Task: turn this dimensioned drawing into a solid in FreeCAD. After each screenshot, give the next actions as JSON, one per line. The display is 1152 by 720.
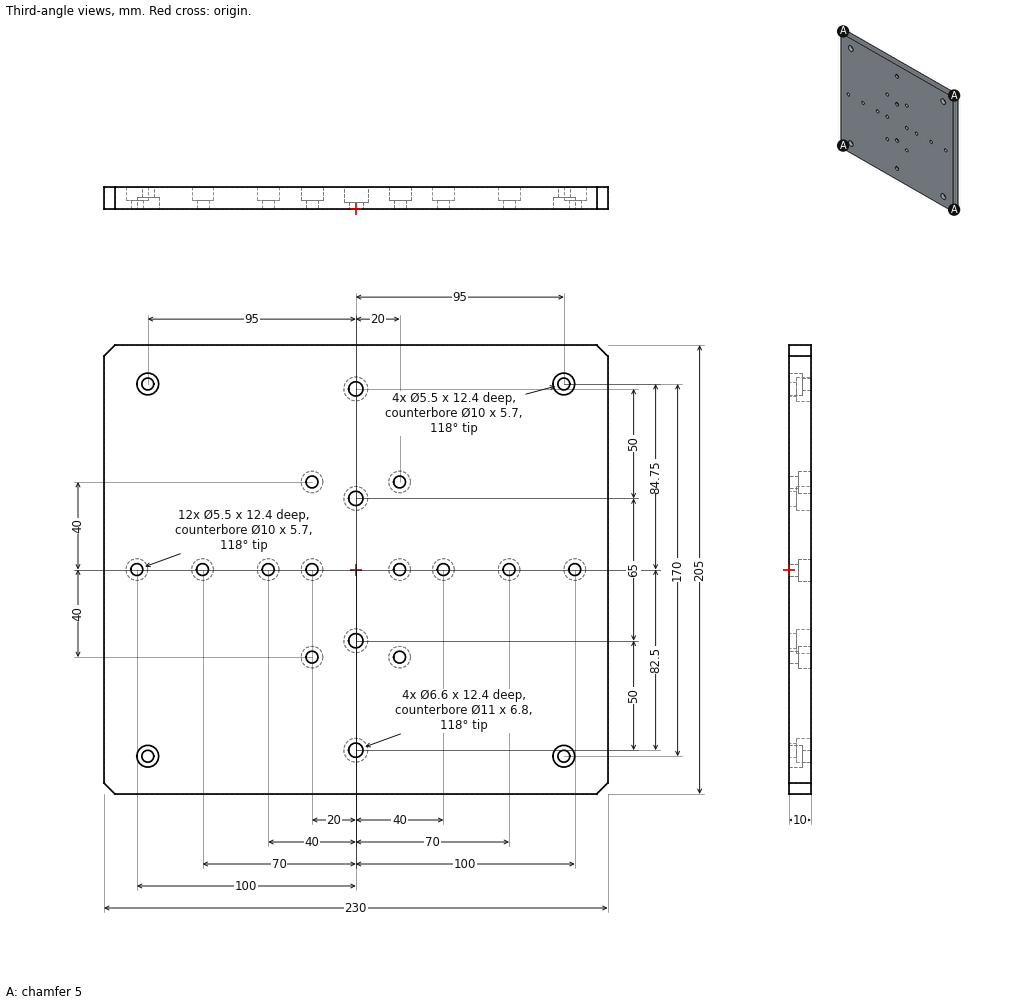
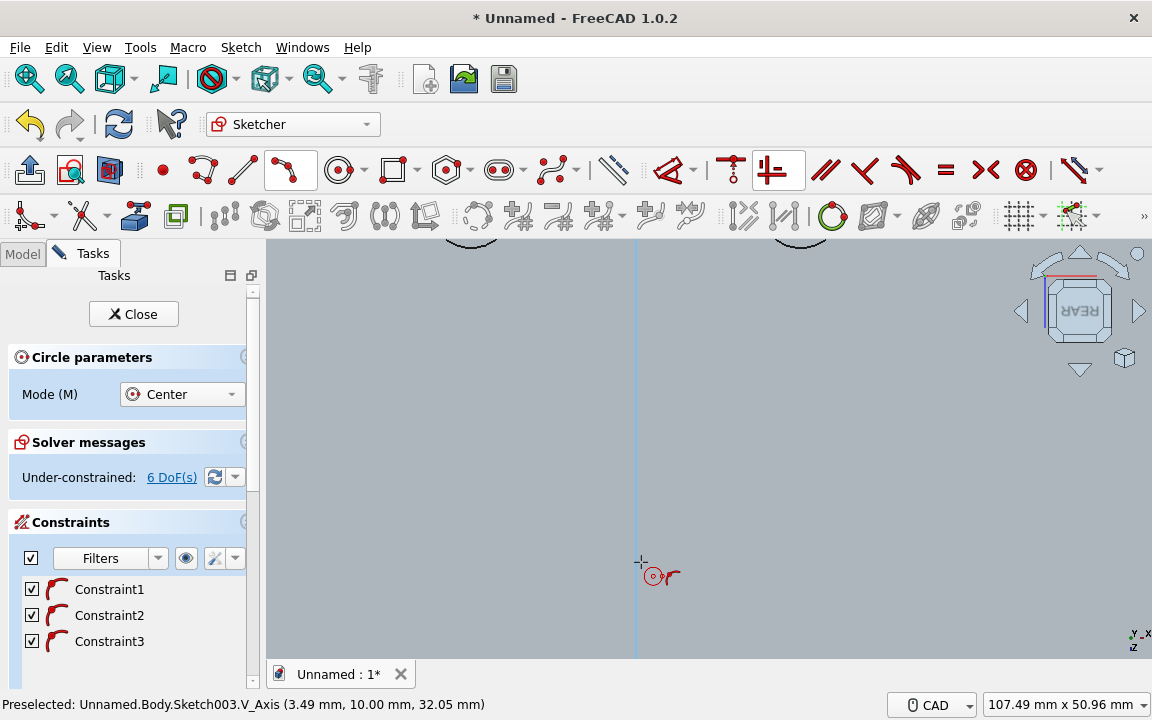
{"action": "scroll", "coordinate": [641, 562], "scroll_direction": "down", "scroll_amount": 9}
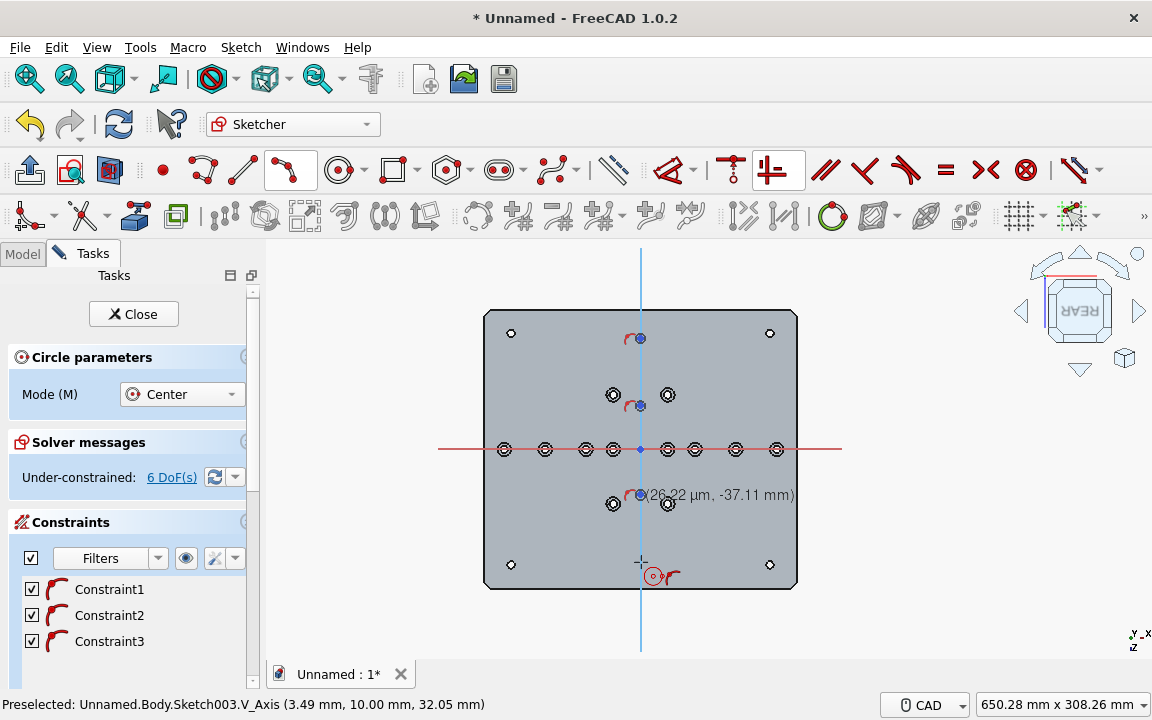
{"action": "left_click", "coordinate": [641, 562]}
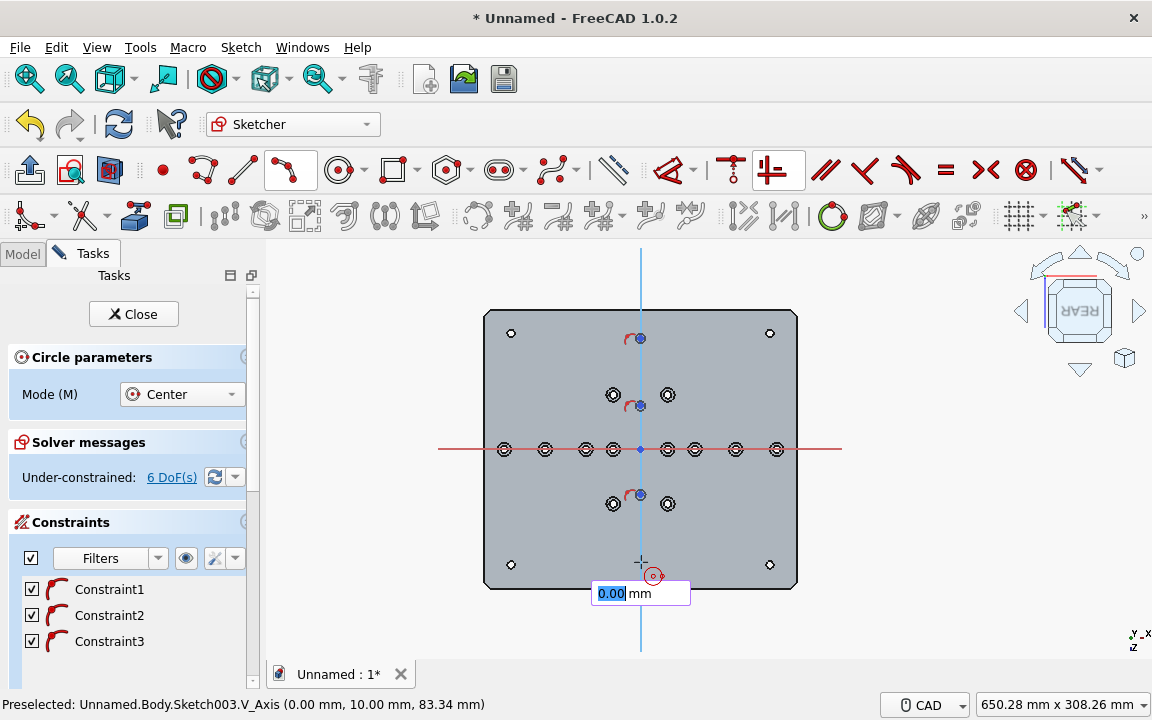
{"action": "scroll", "coordinate": [645, 560], "scroll_direction": "up", "scroll_amount": 7}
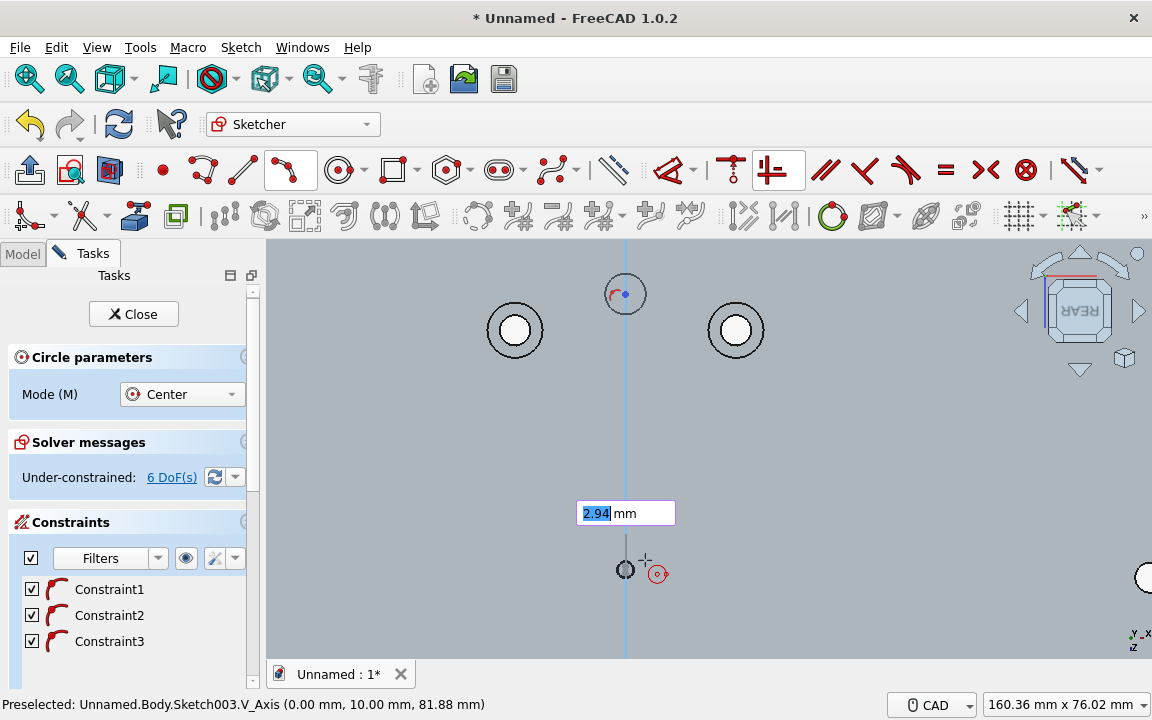
{"action": "left_click", "coordinate": [643, 559]}
{"action": "key", "text": "Escape"}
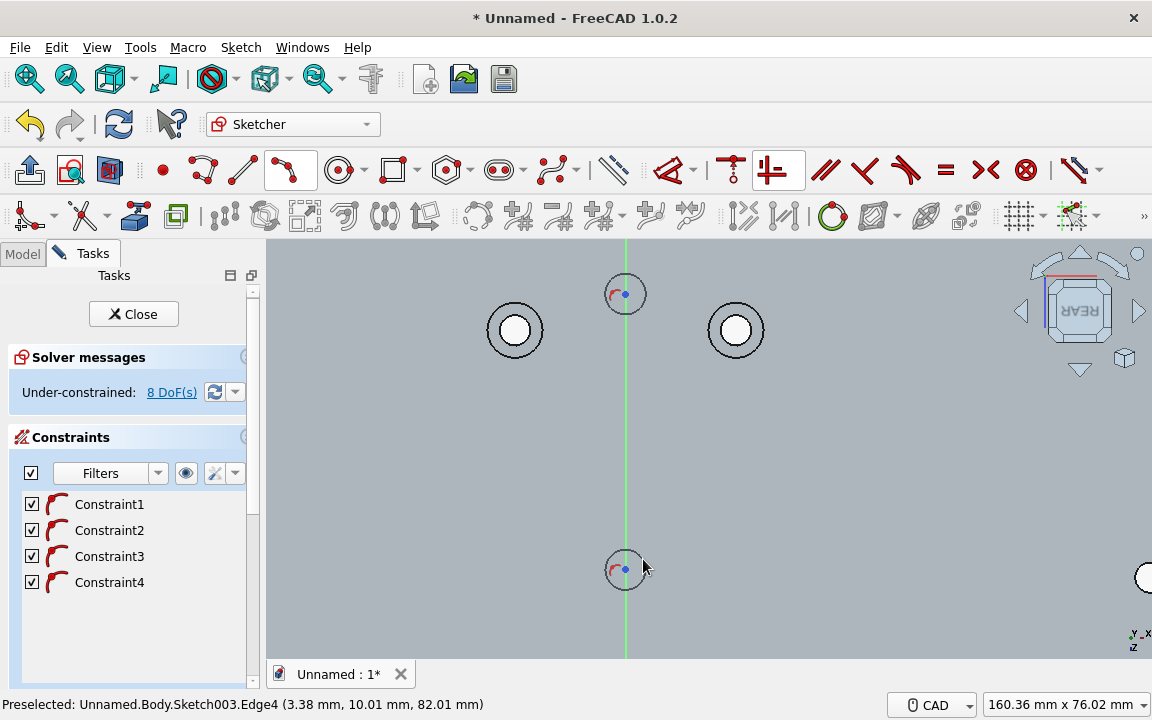
{"action": "scroll", "coordinate": [645, 560], "scroll_direction": "down", "scroll_amount": 7}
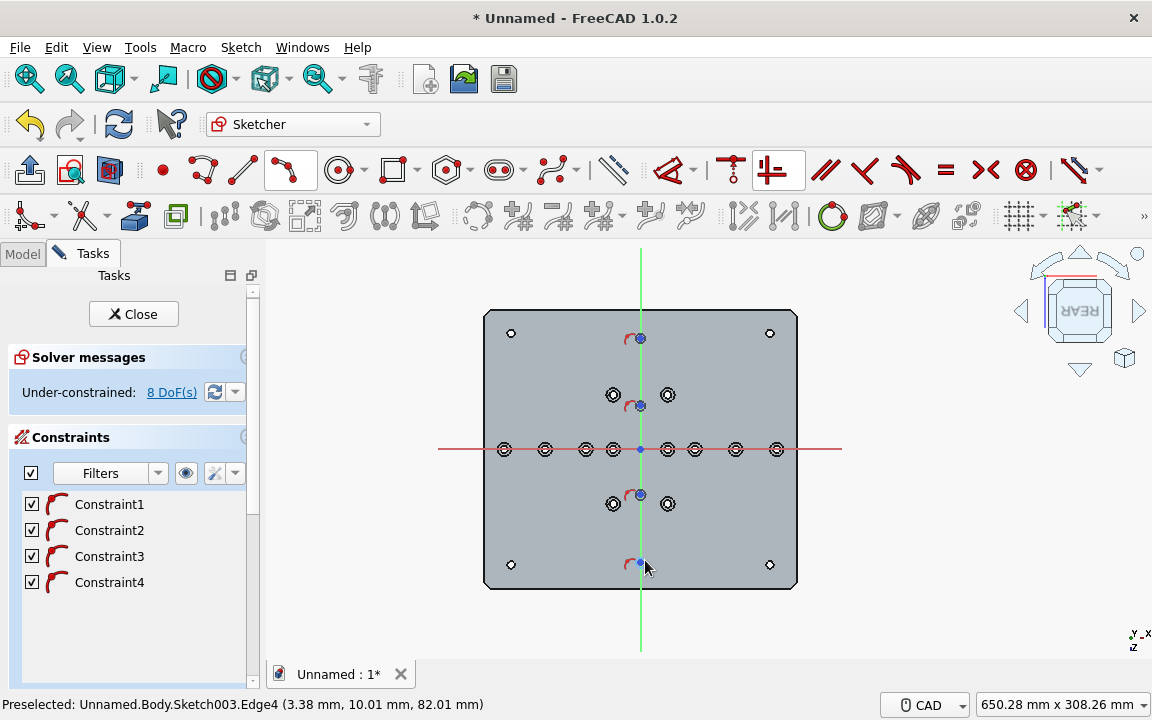
{"action": "scroll", "coordinate": [644, 335], "scroll_direction": "up", "scroll_amount": 7}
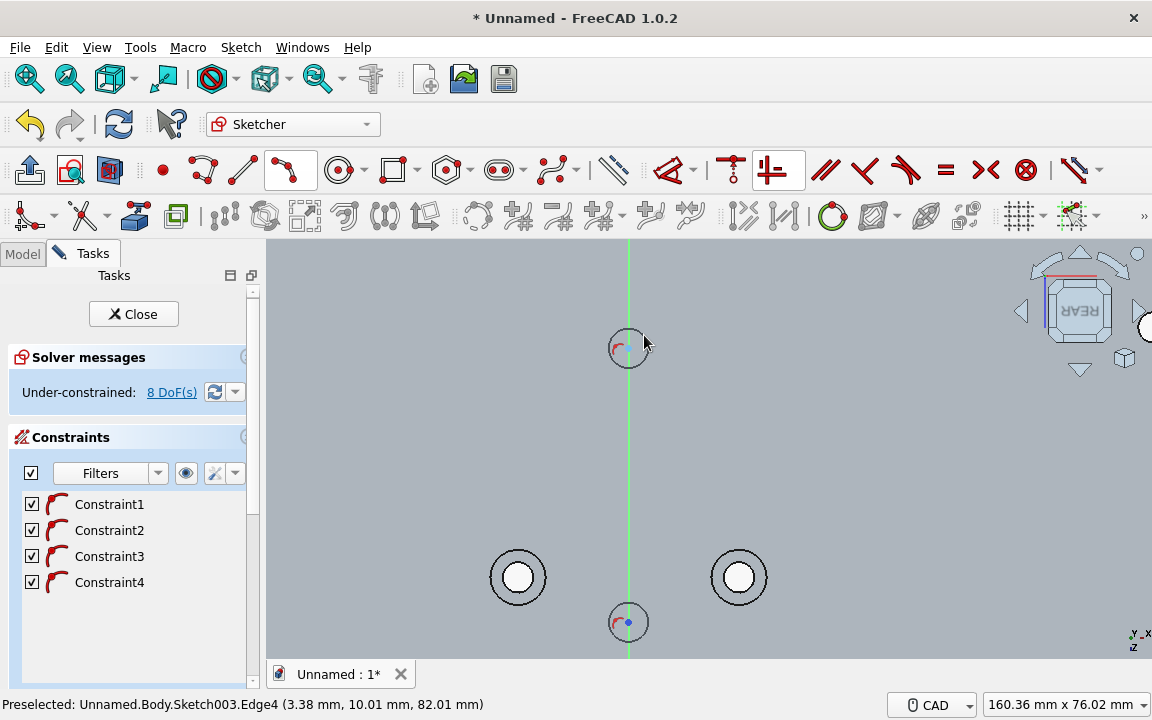
{"action": "left_click", "coordinate": [642, 334]}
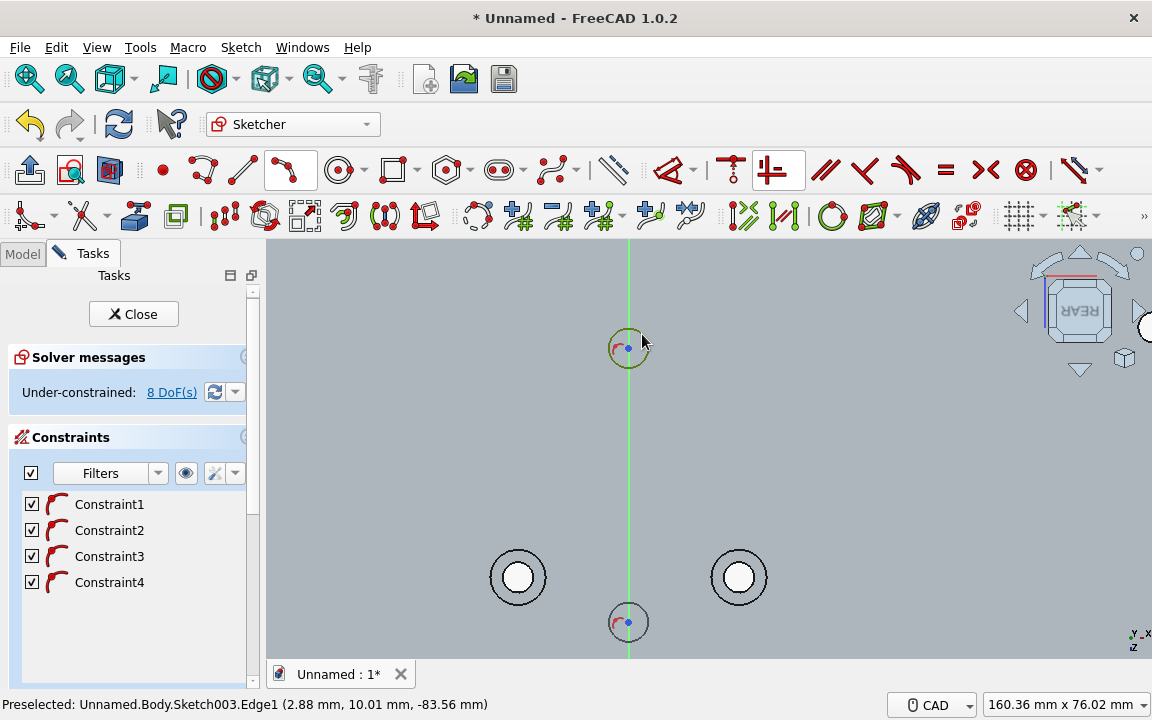
{"action": "left_click", "coordinate": [642, 608]}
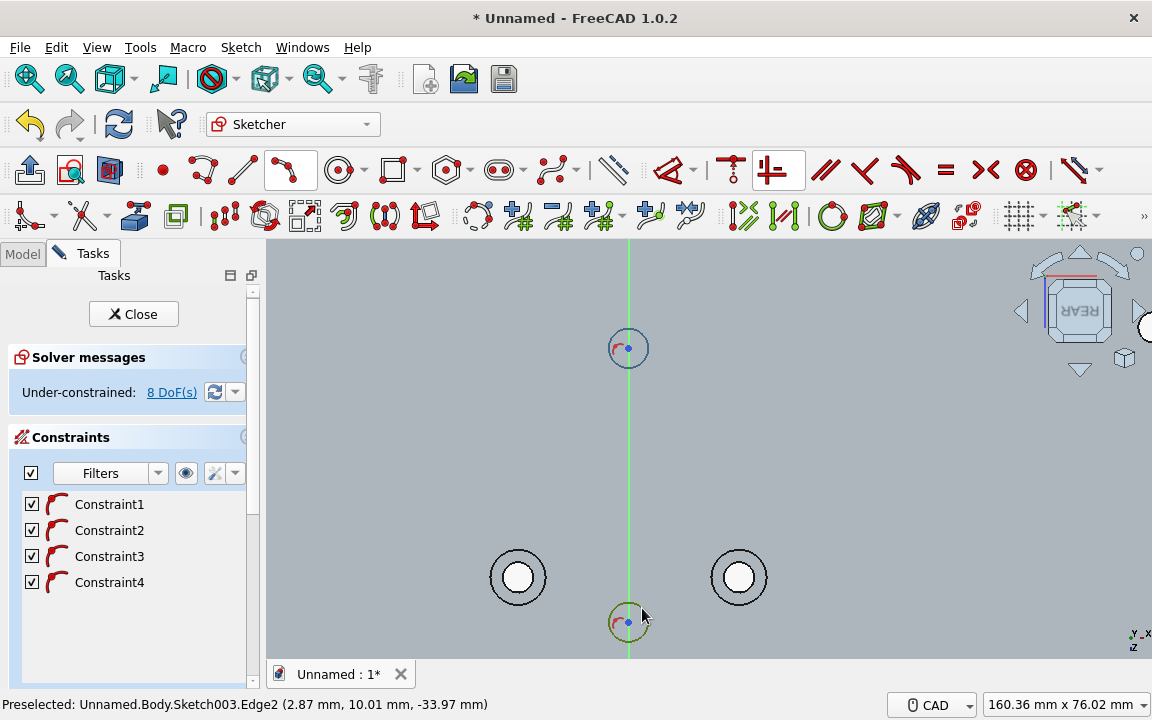
{"action": "scroll", "coordinate": [644, 335], "scroll_direction": "down", "scroll_amount": 7}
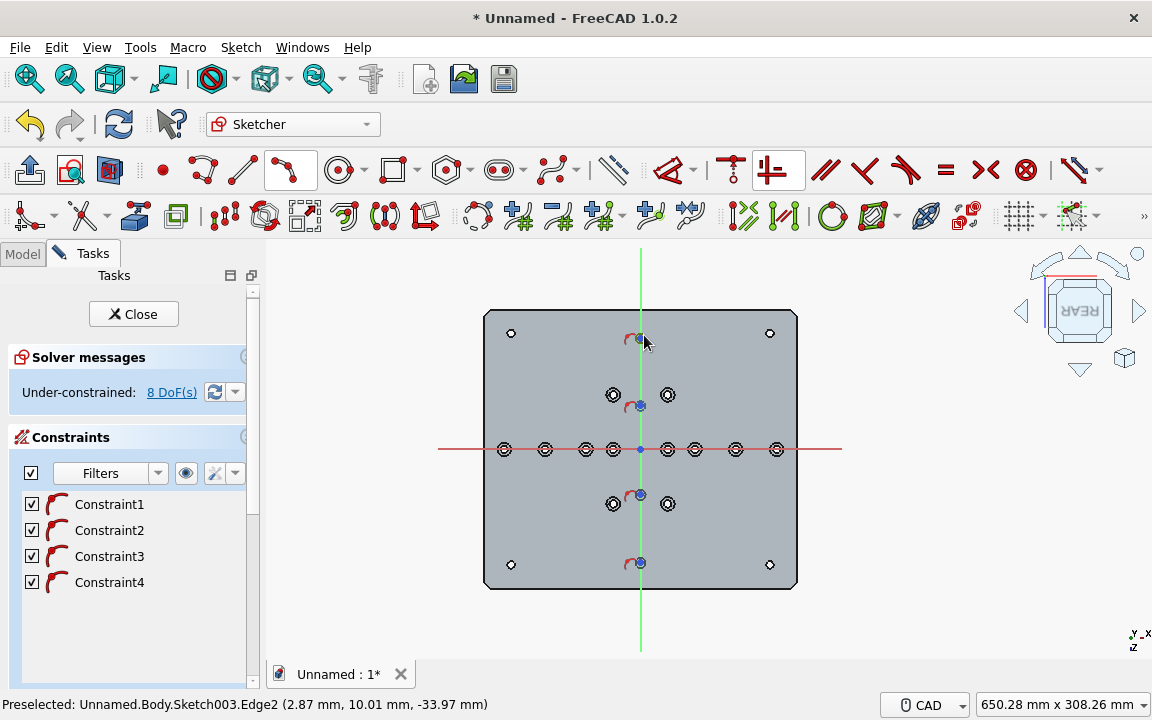
{"action": "scroll", "coordinate": [644, 491], "scroll_direction": "up", "scroll_amount": 7}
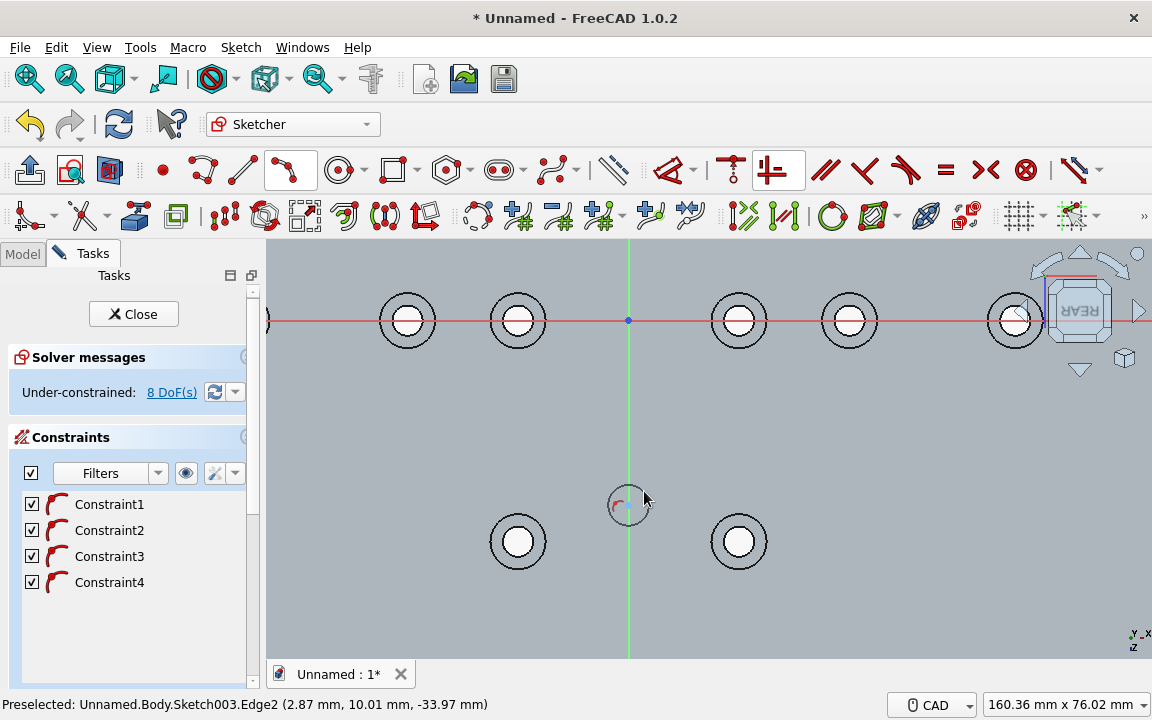
{"action": "left_click", "coordinate": [643, 491]}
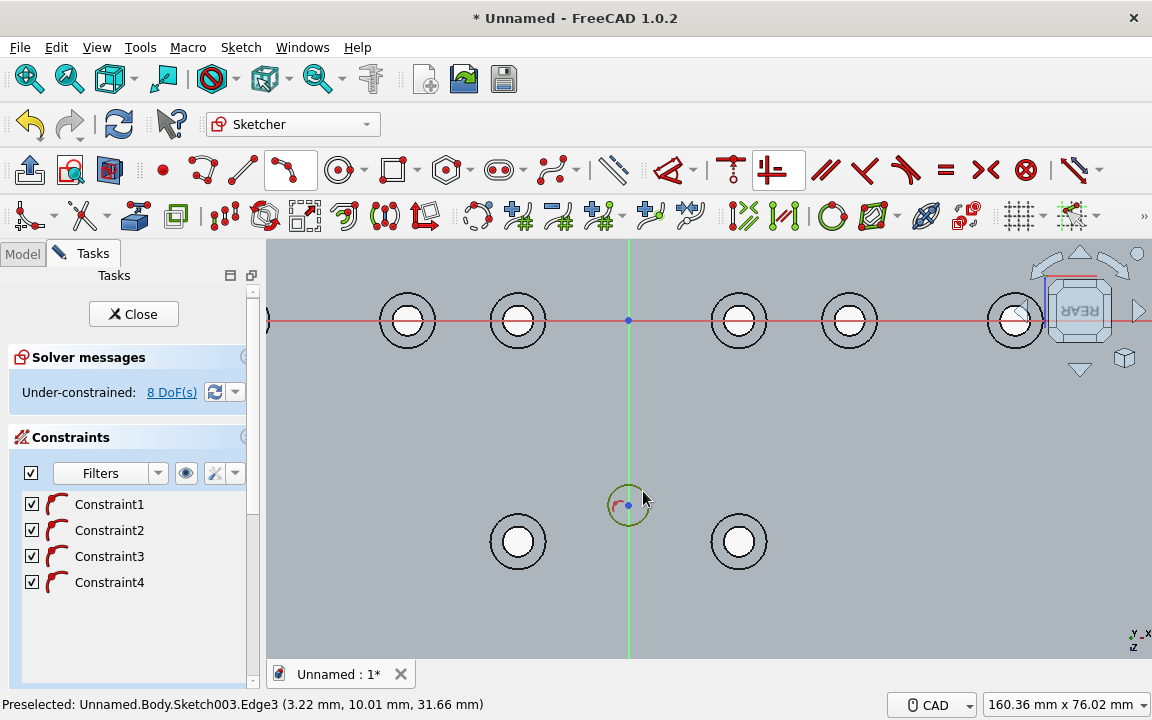
{"action": "scroll", "coordinate": [644, 491], "scroll_direction": "down", "scroll_amount": 7}